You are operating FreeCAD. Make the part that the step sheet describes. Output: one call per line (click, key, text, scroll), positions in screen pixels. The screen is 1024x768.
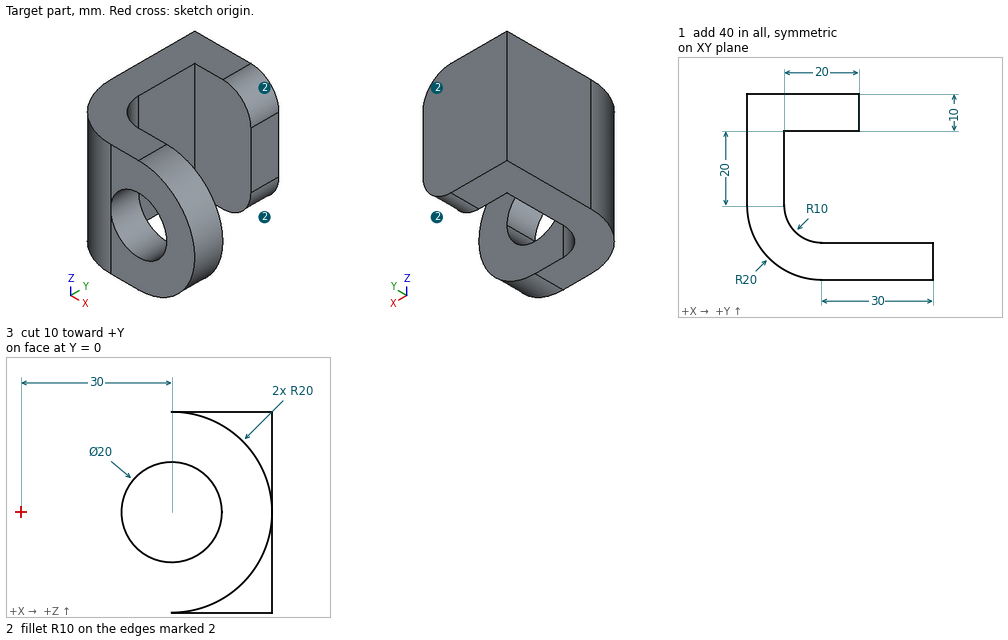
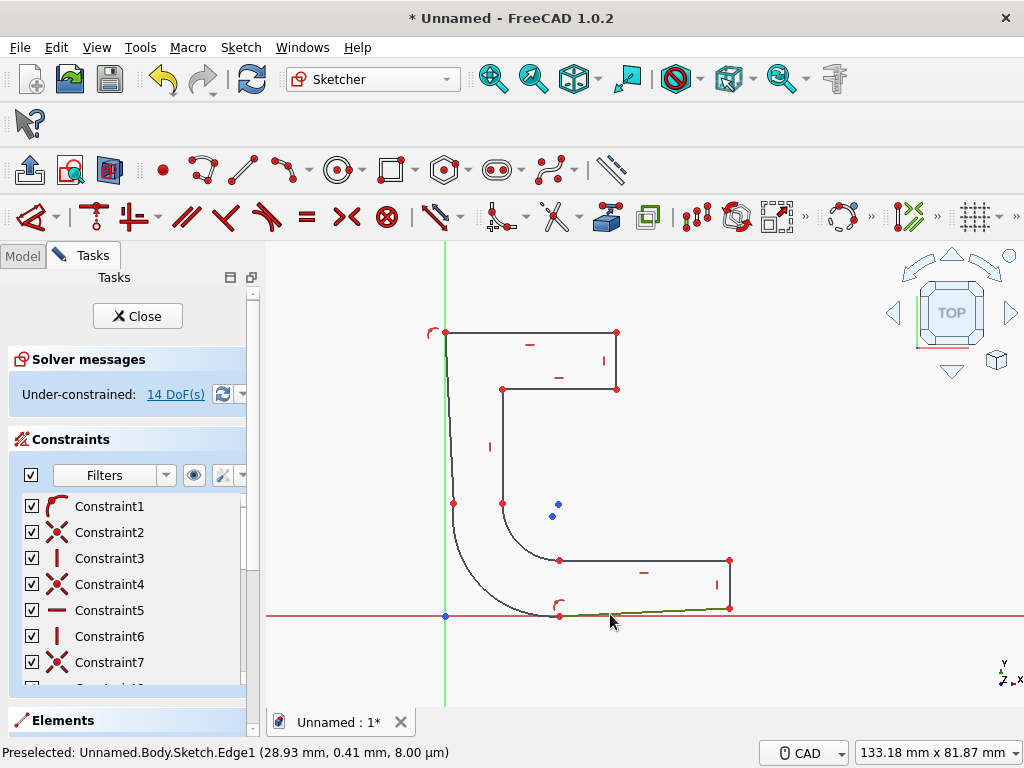
click(461, 556)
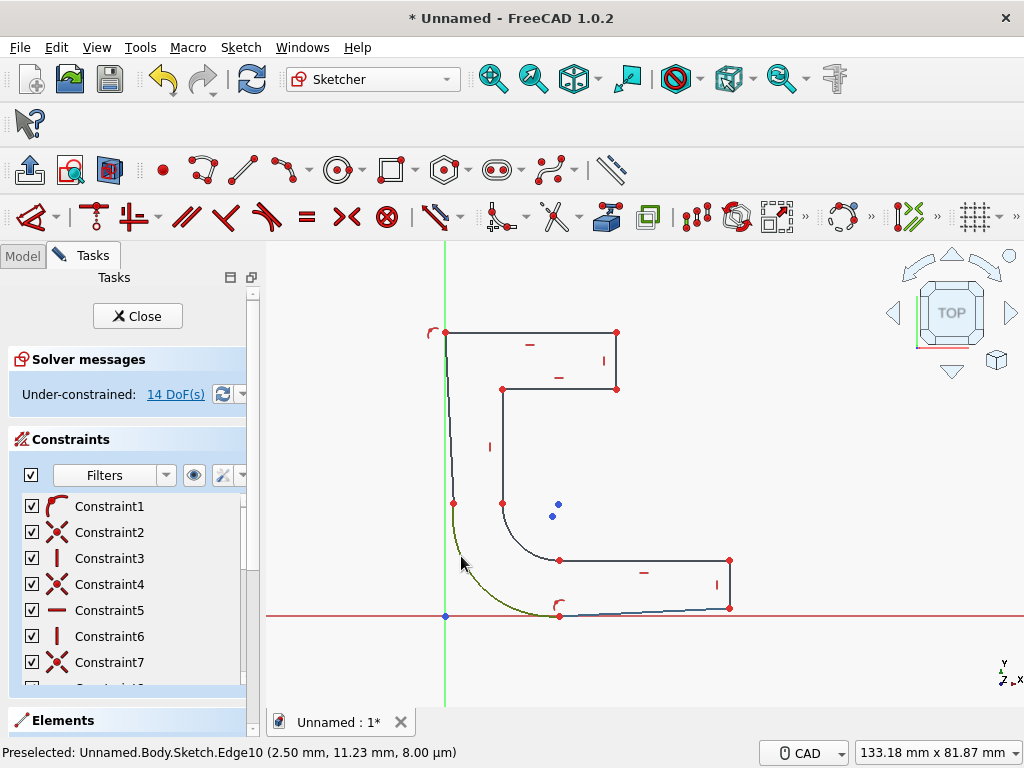
click(268, 218)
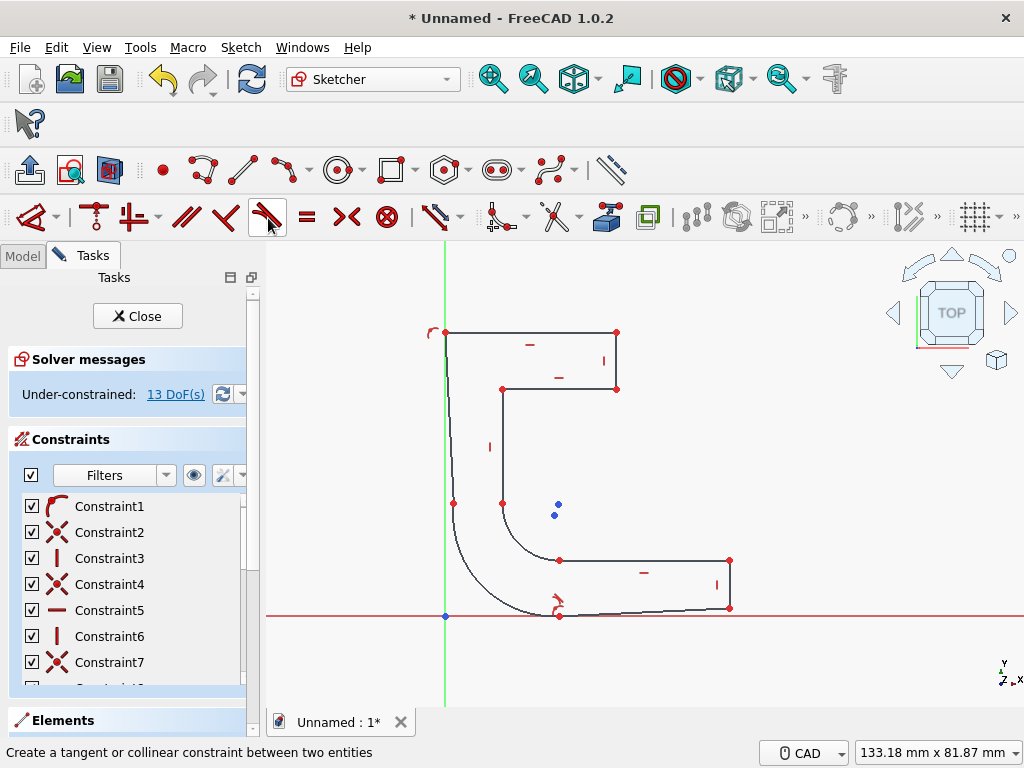
click(679, 561)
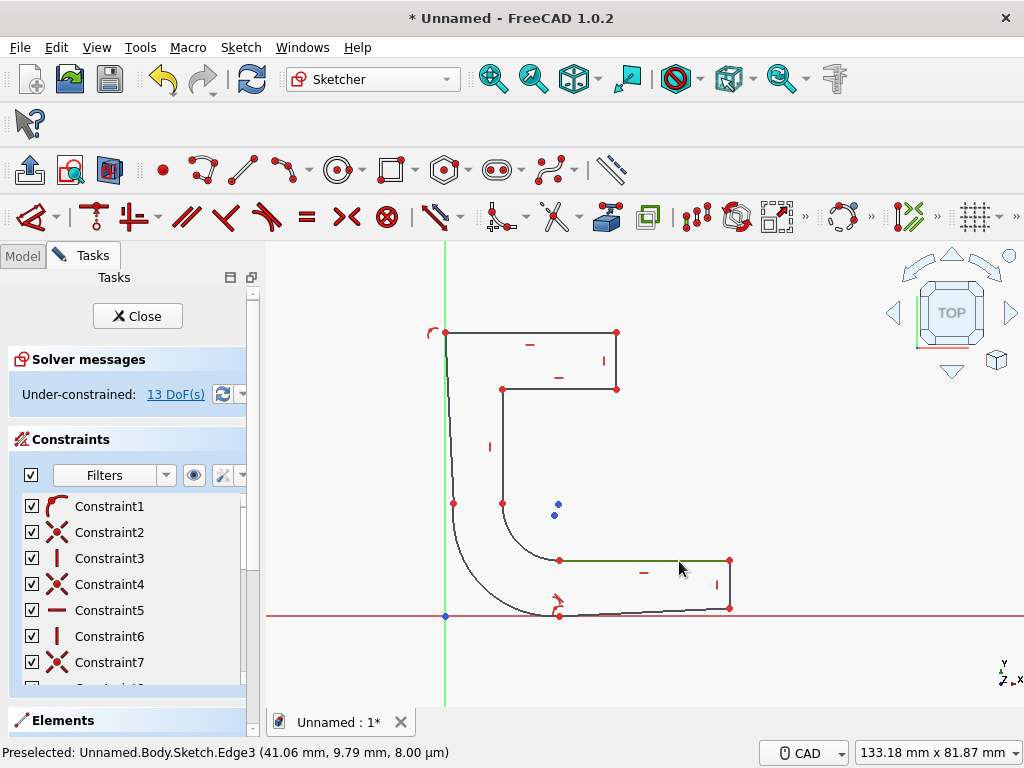
click(509, 530)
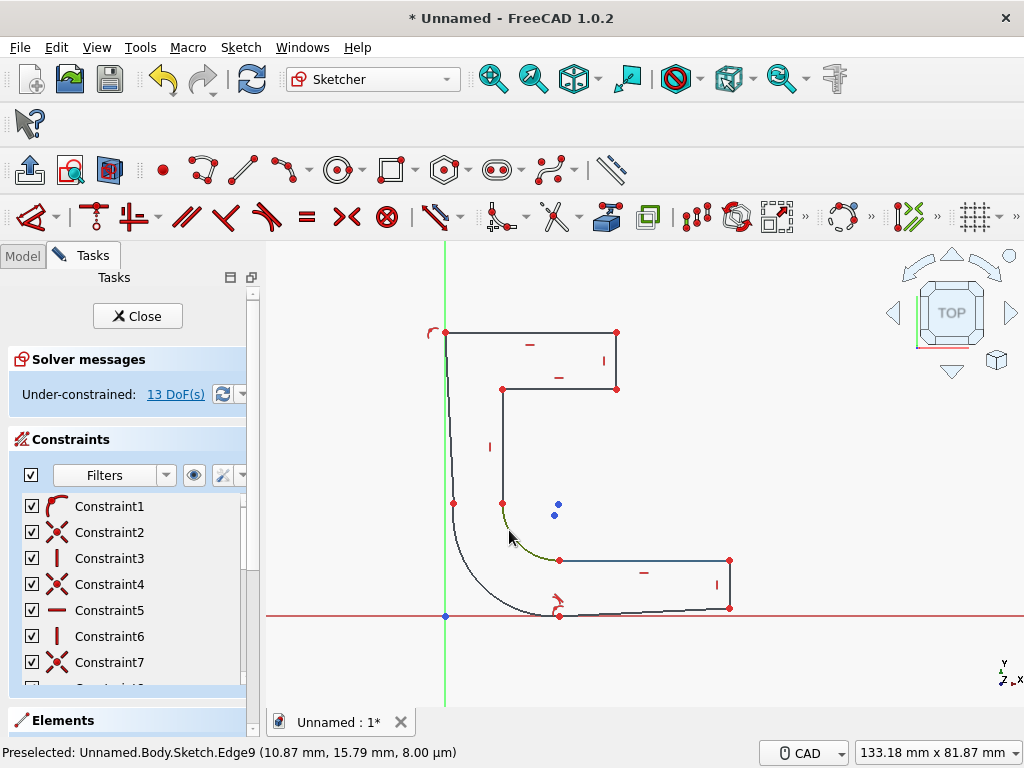
click(268, 218)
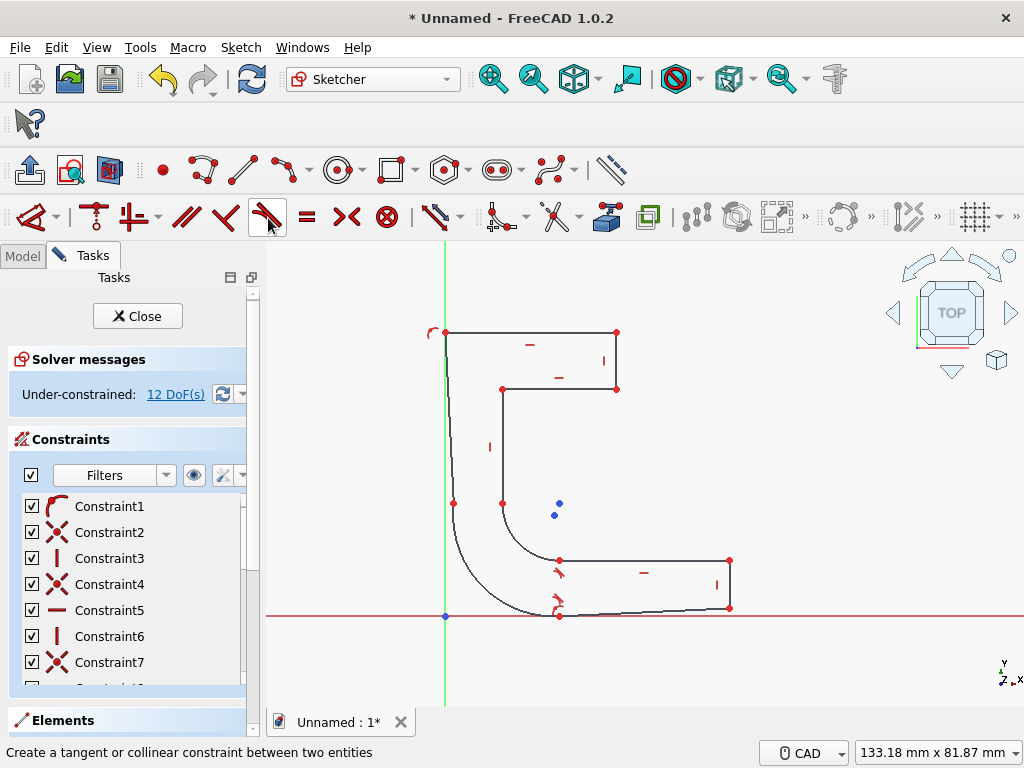
click(503, 470)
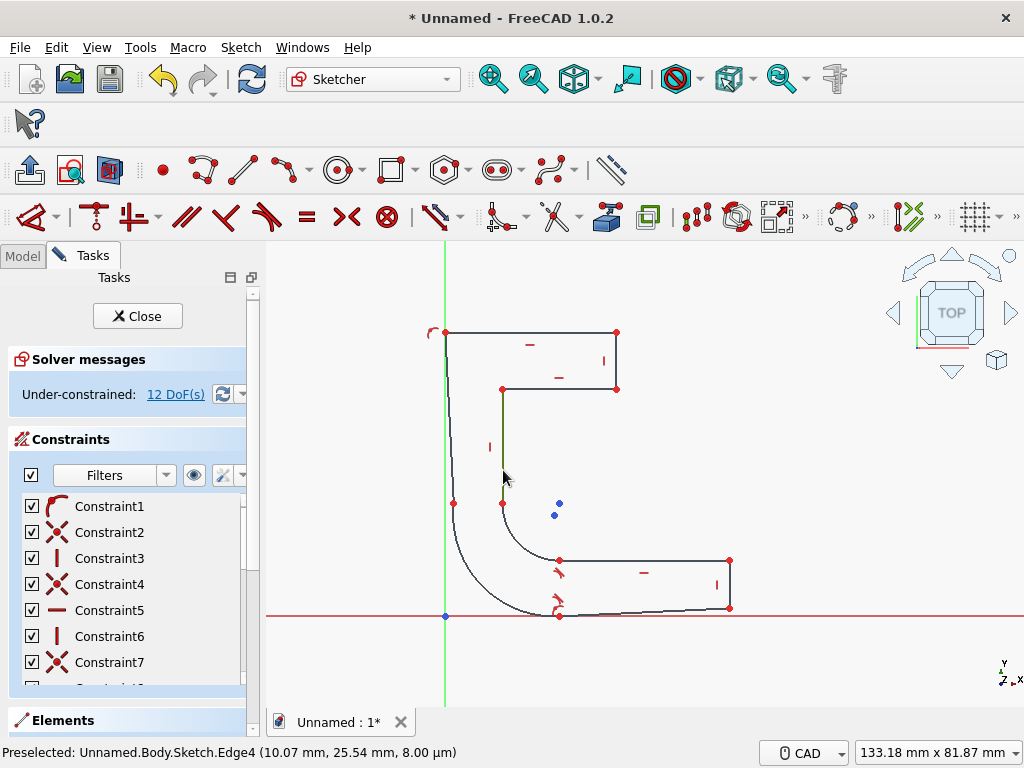
click(509, 530)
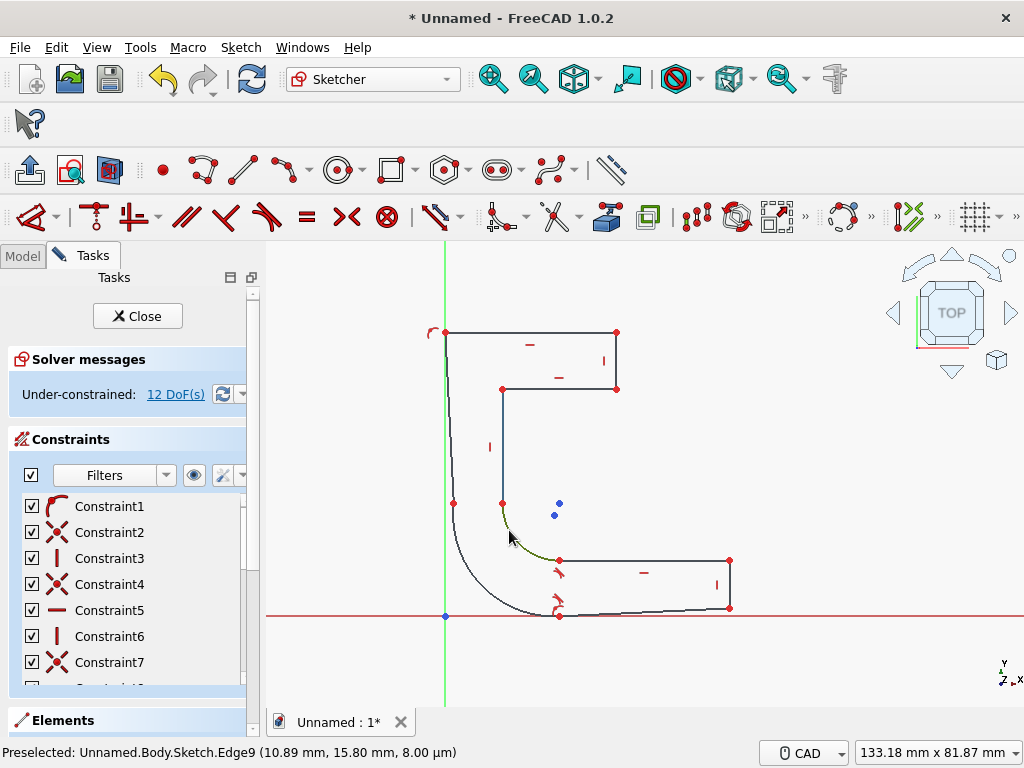
key(t)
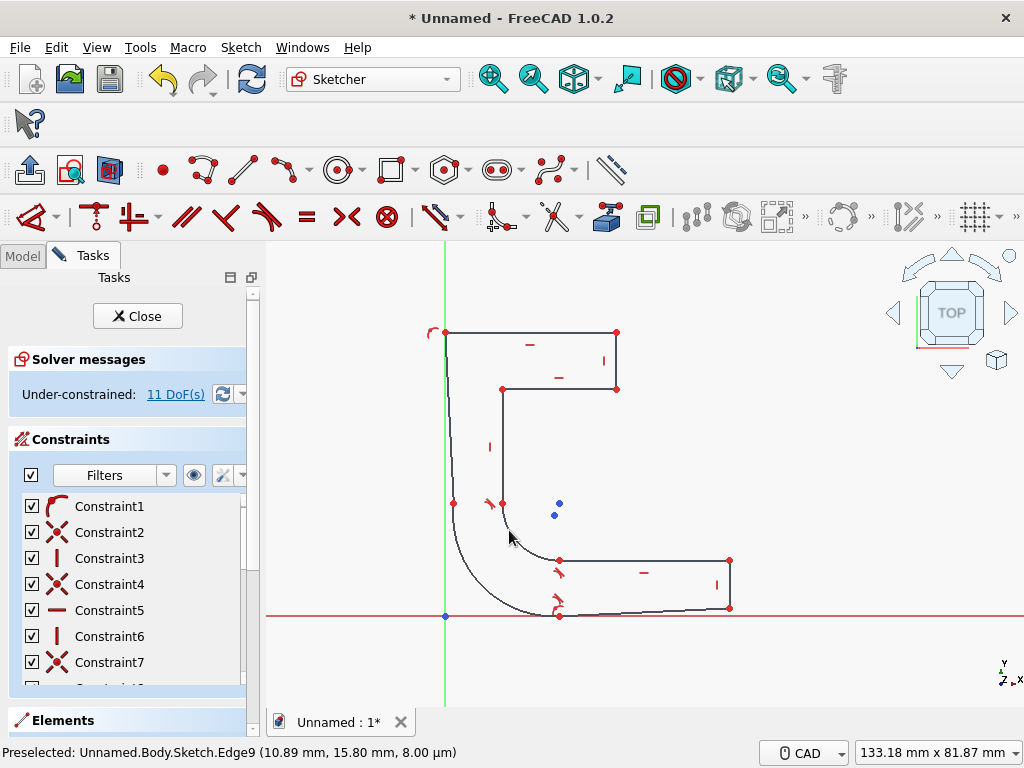
click(448, 384)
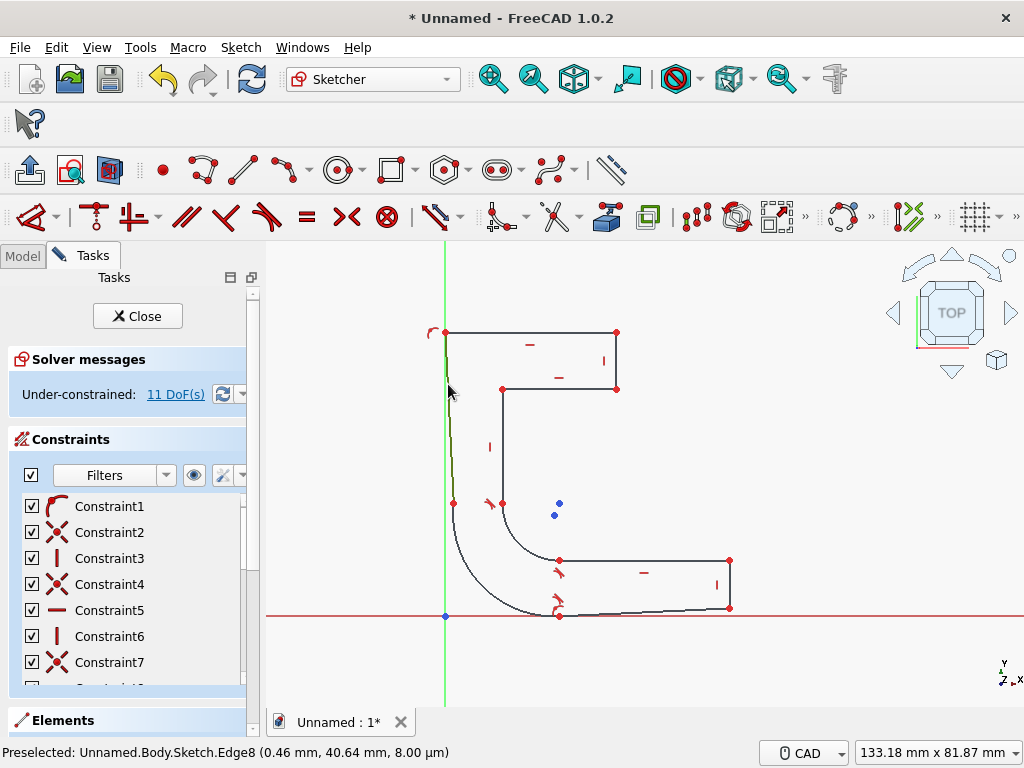
click(462, 555)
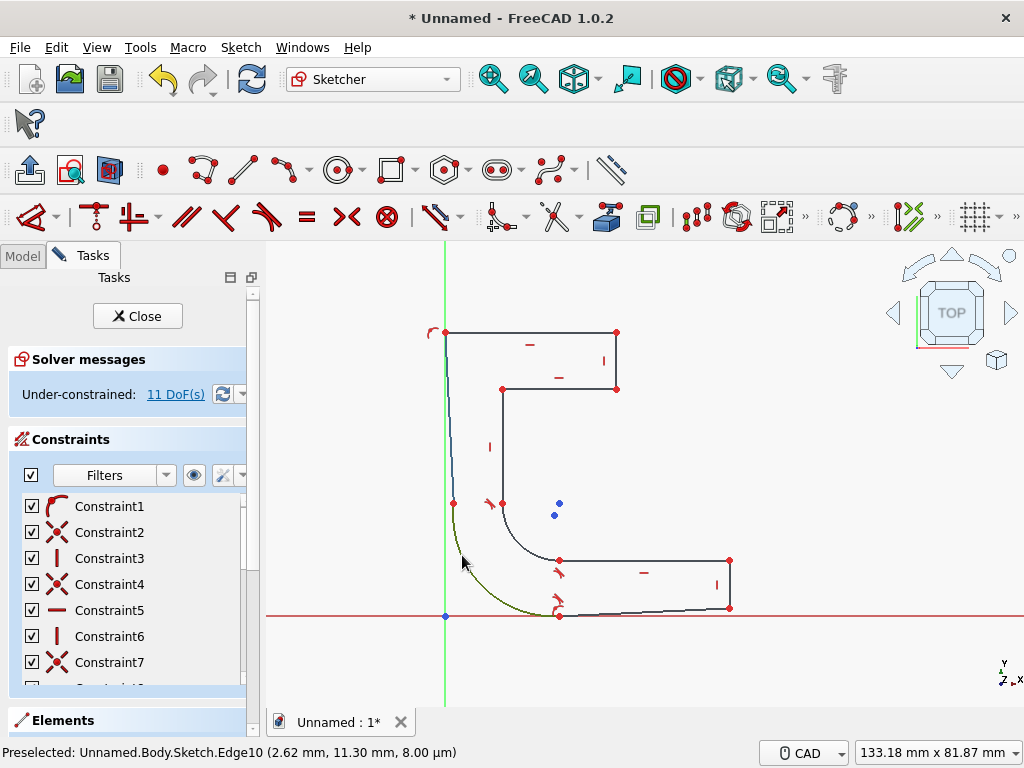
click(268, 218)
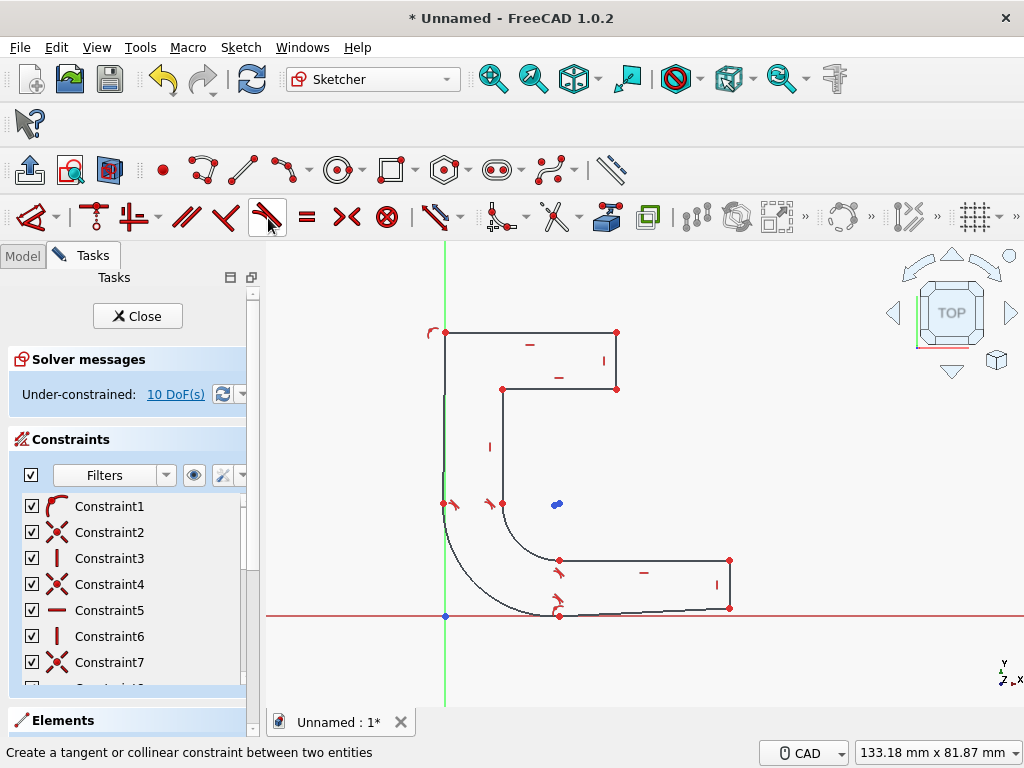
click(610, 614)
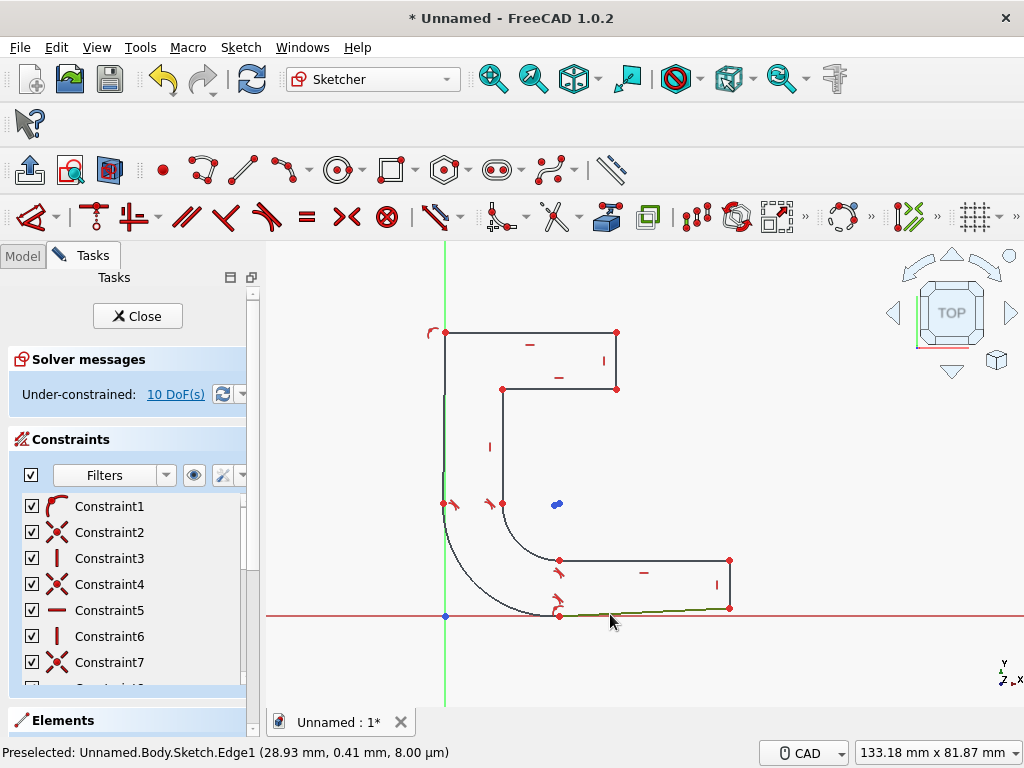
click(160, 218)